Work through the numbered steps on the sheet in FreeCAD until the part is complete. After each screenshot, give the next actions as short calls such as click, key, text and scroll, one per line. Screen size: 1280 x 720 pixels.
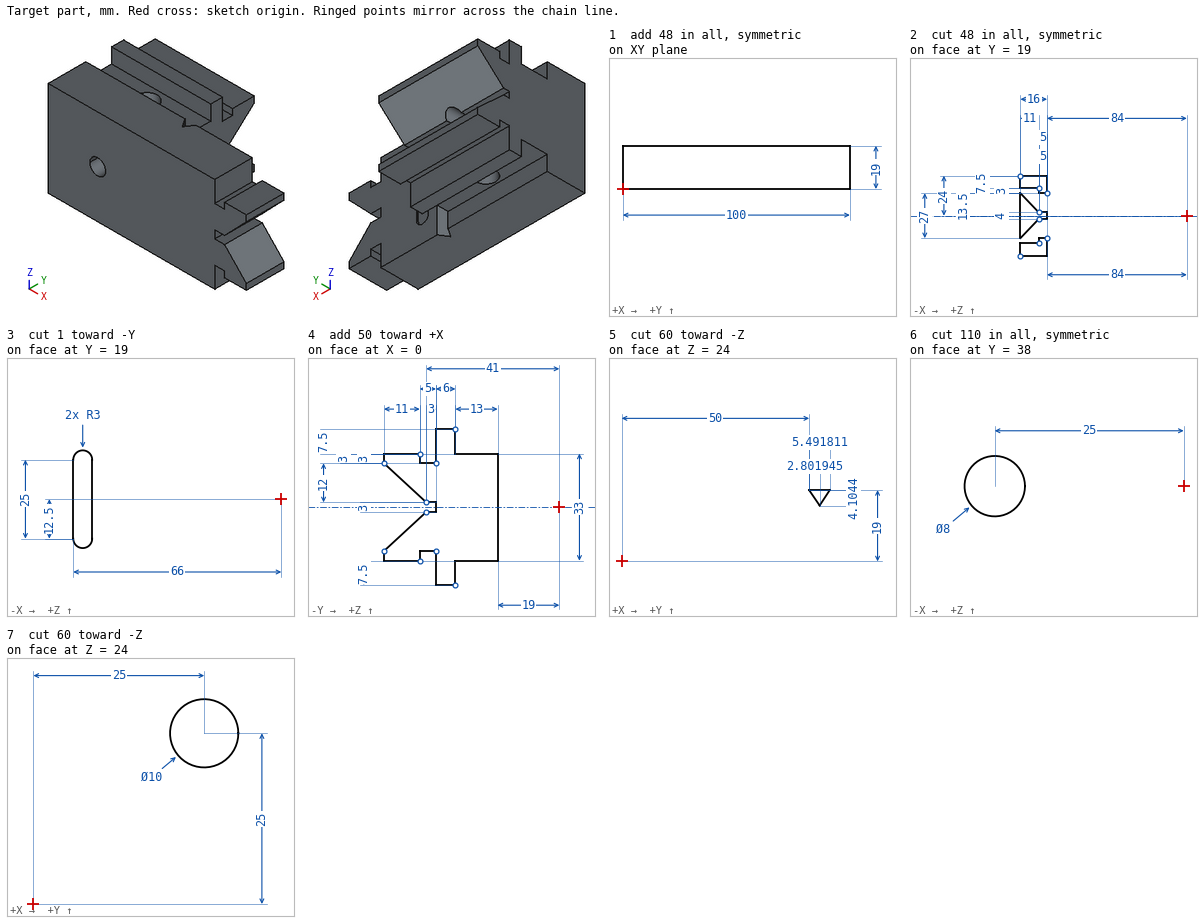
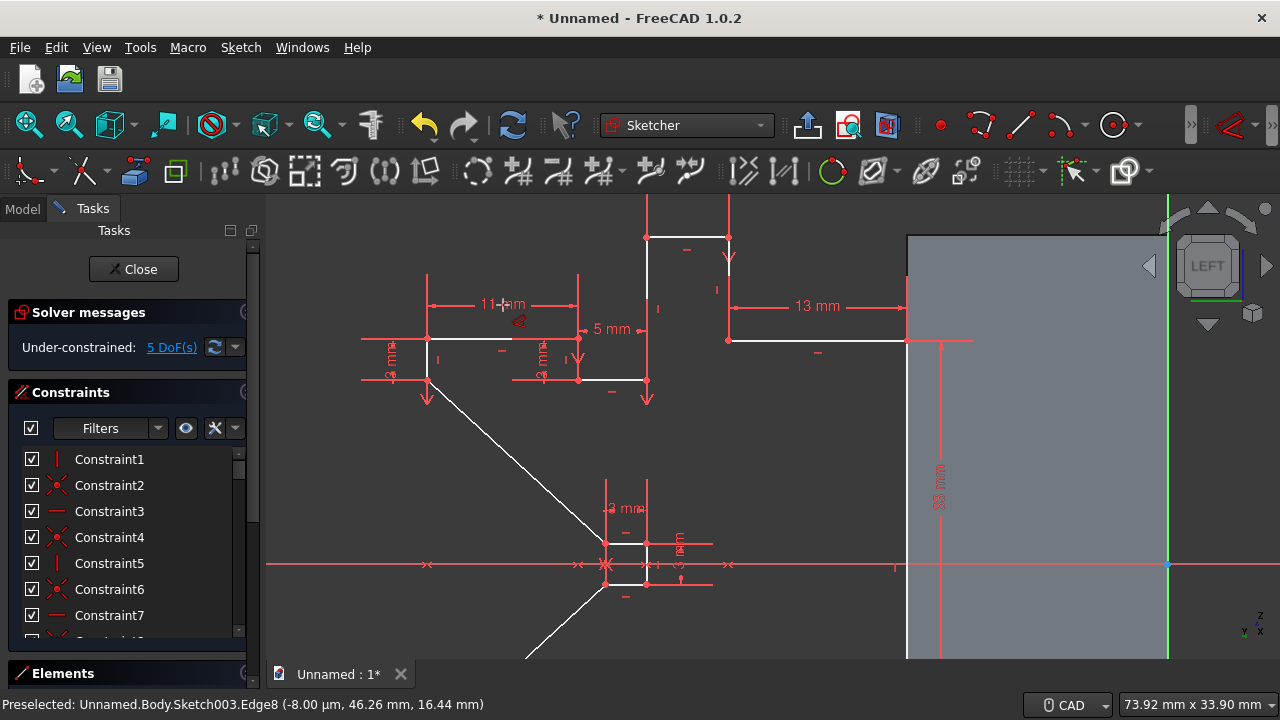
click(729, 310)
click(695, 289)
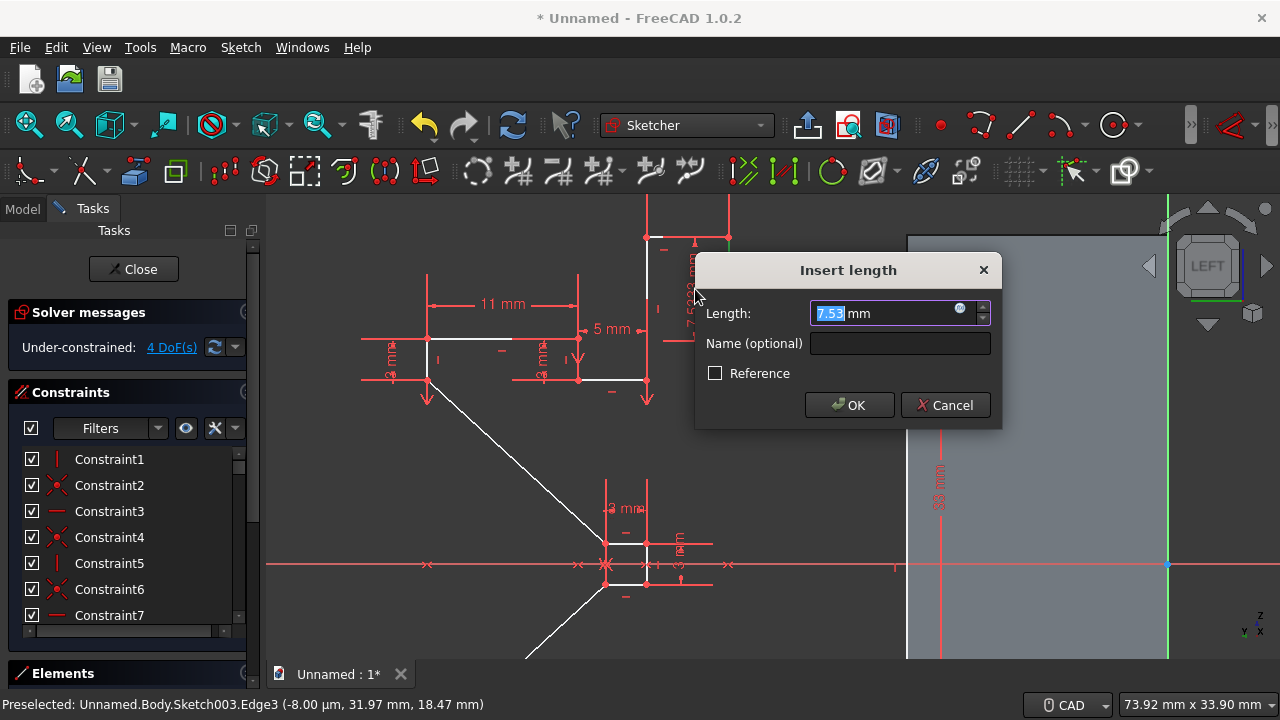
text(7.5)
key(Return)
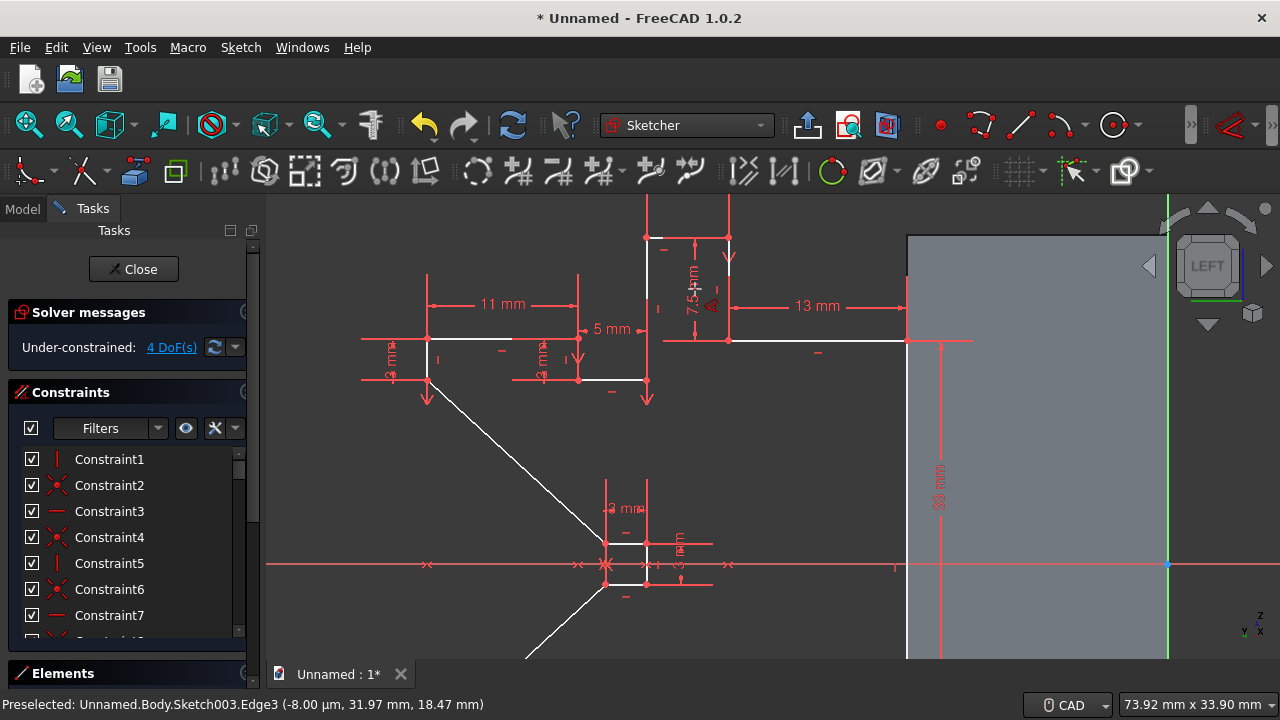
scroll(629, 314, down, 4)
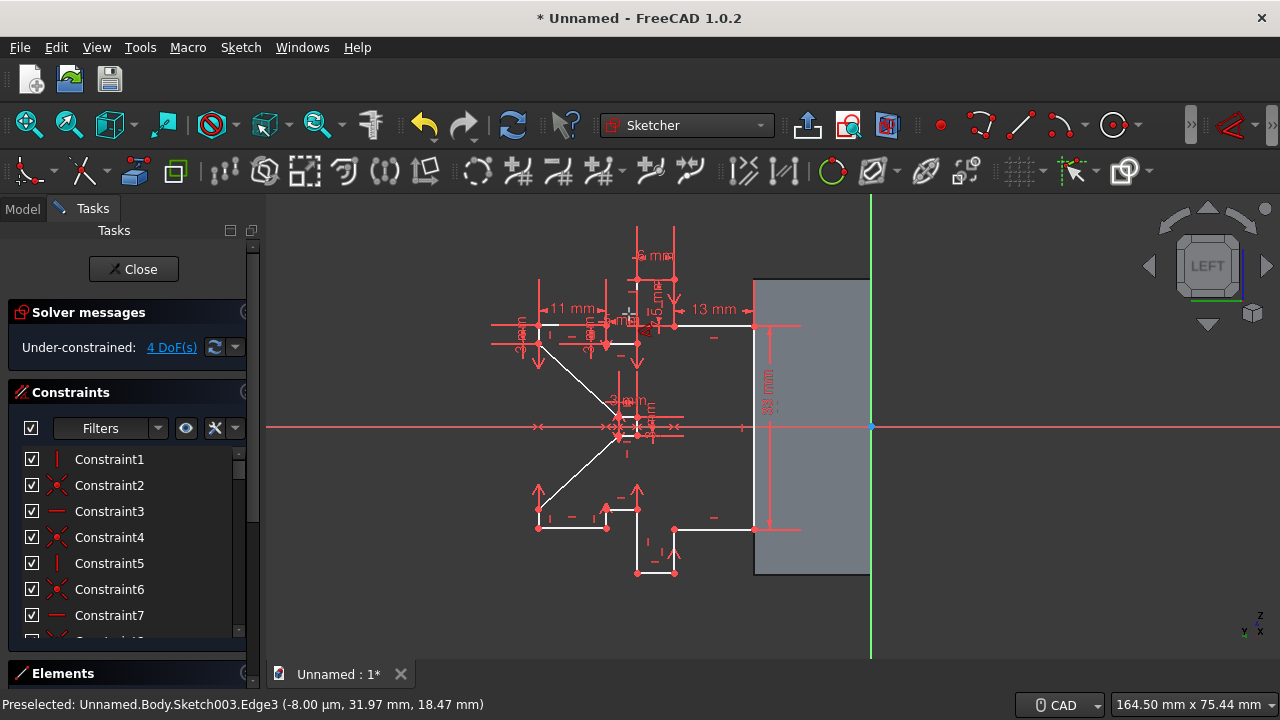
click(674, 560)
click(708, 551)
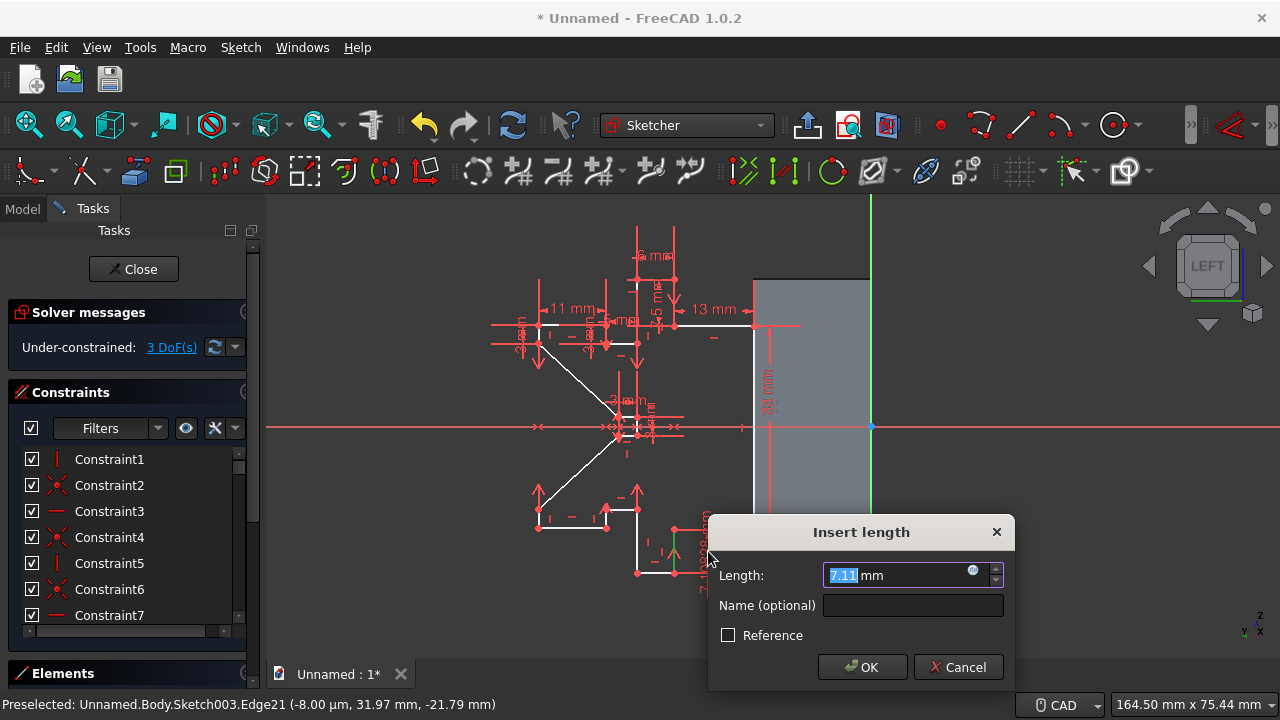
text(7.5)
key(Return)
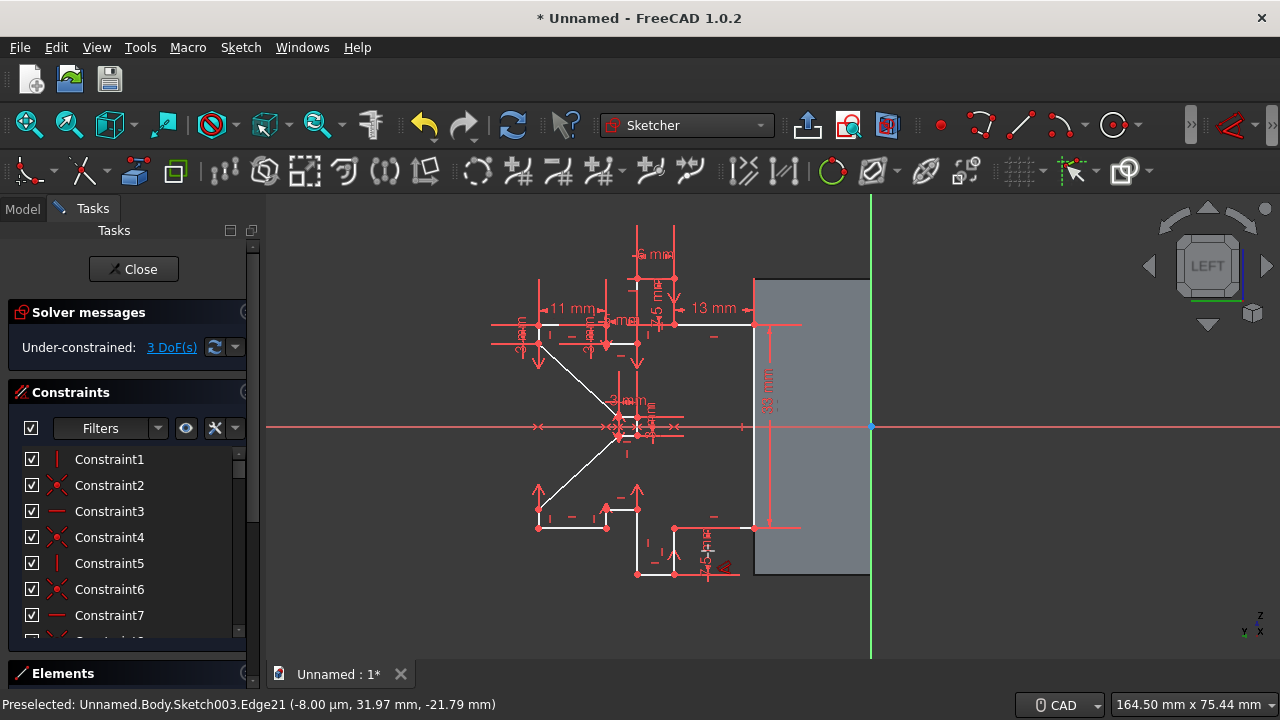
click(754, 528)
click(813, 562)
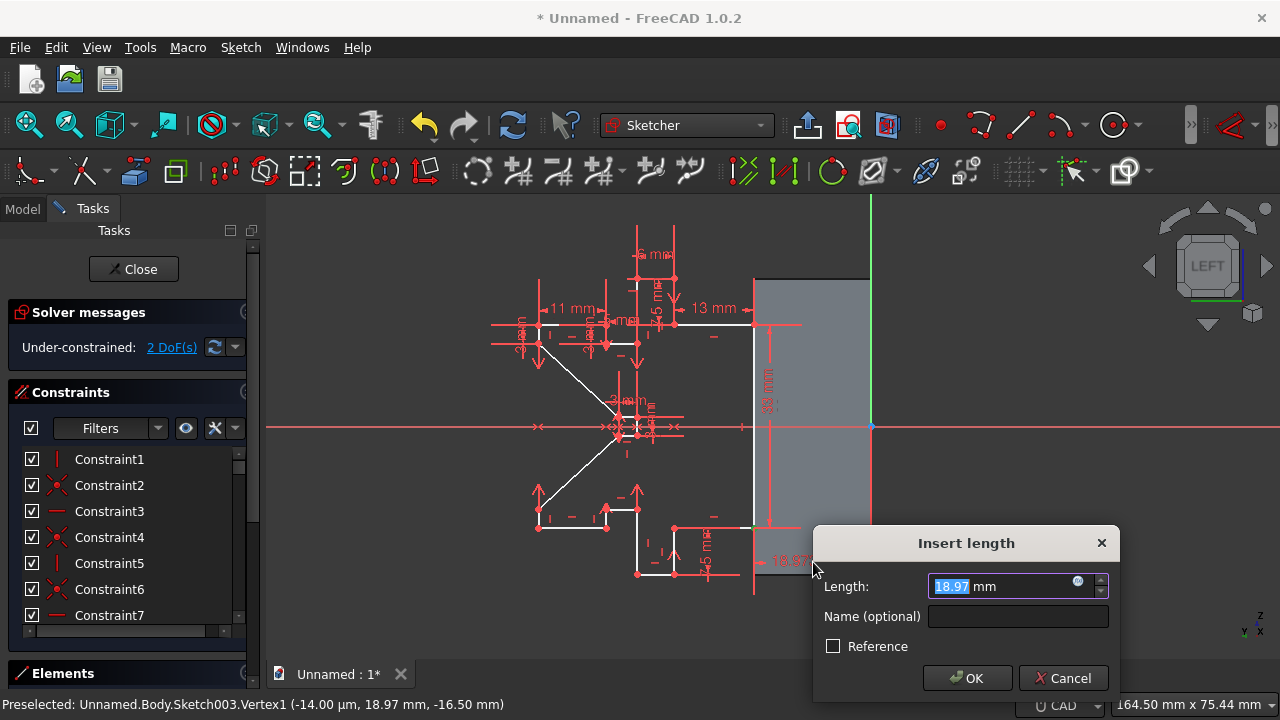
text(19)
key(Return)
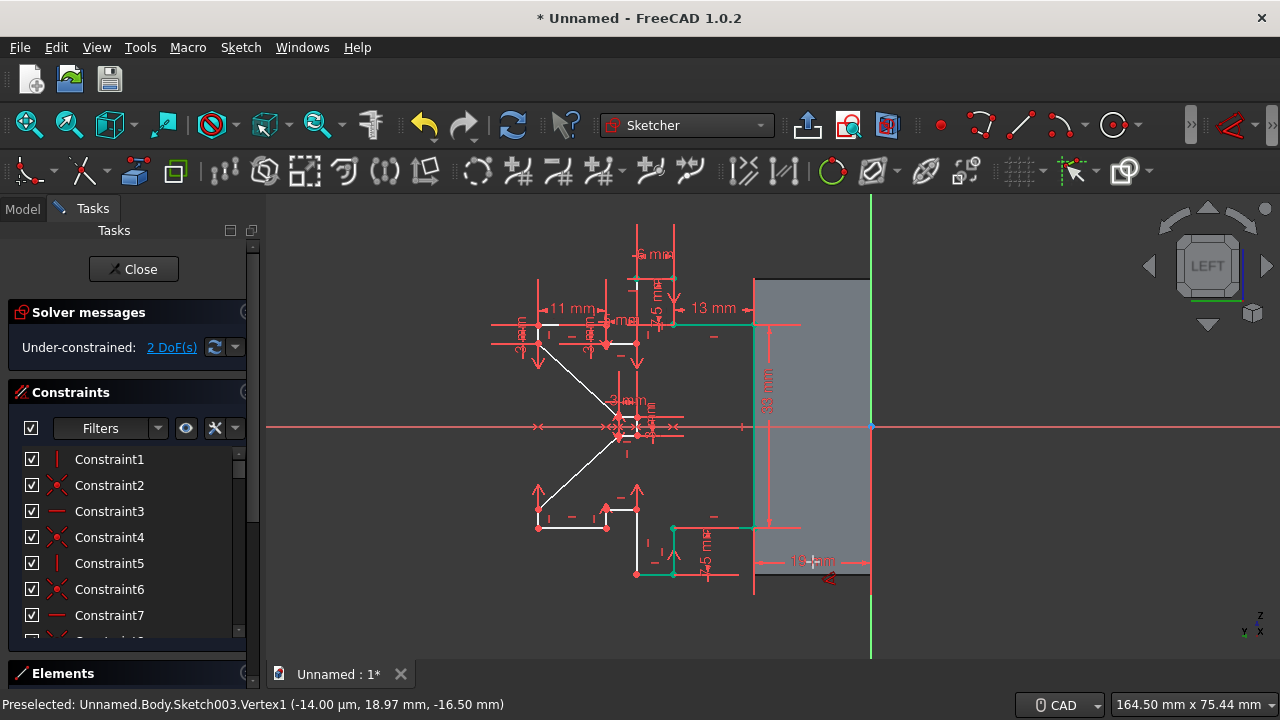
click(619, 417)
click(687, 461)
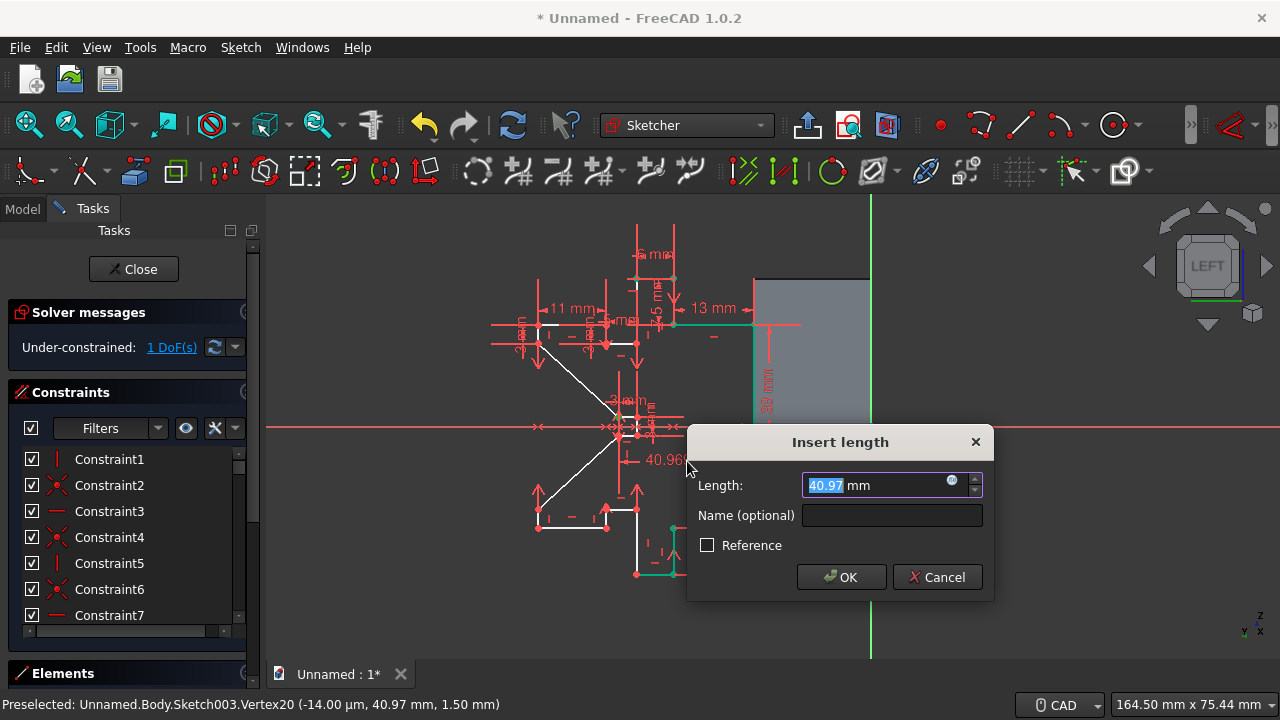
text(41)
key(Return)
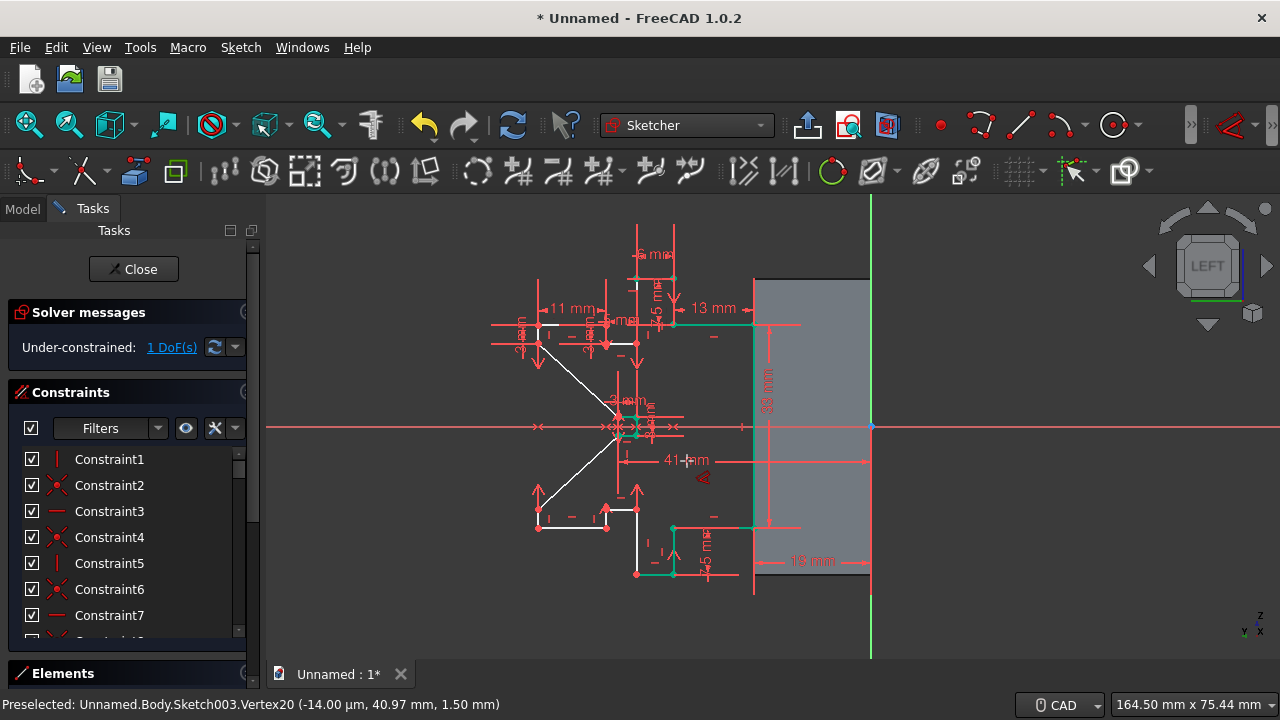
click(562, 366)
click(504, 381)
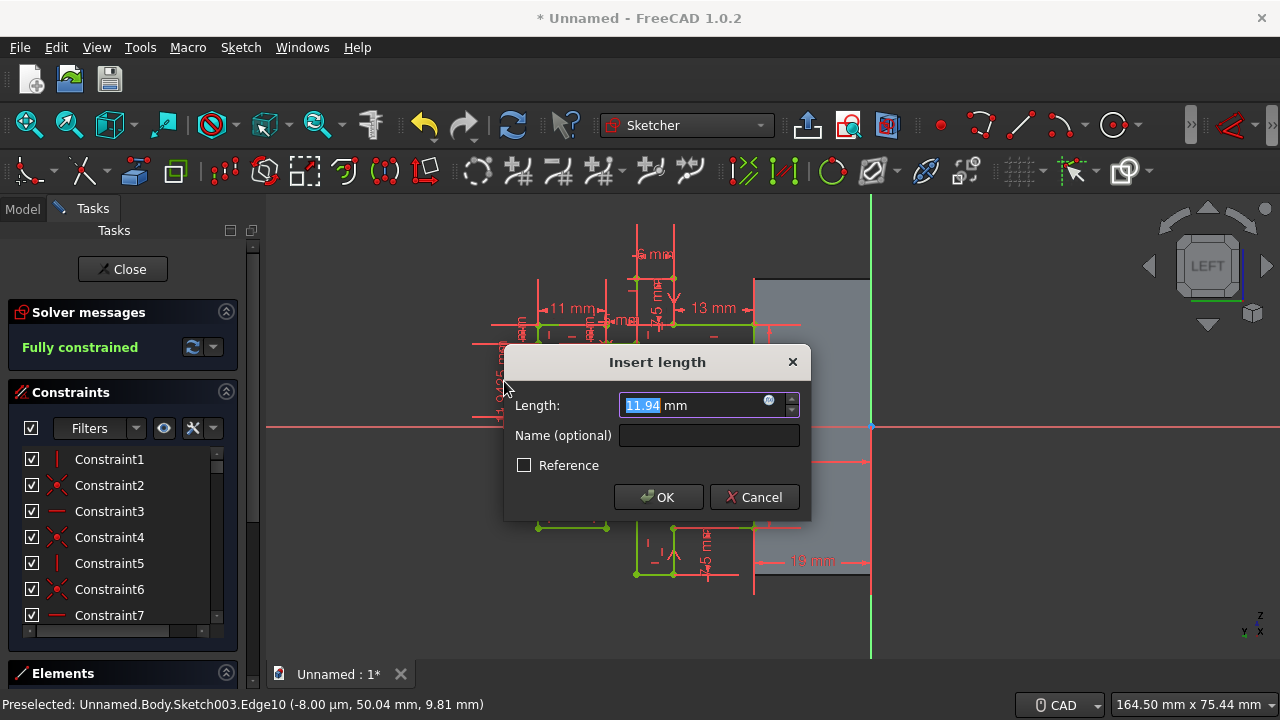
text(12)
key(Return)
key(Escape)